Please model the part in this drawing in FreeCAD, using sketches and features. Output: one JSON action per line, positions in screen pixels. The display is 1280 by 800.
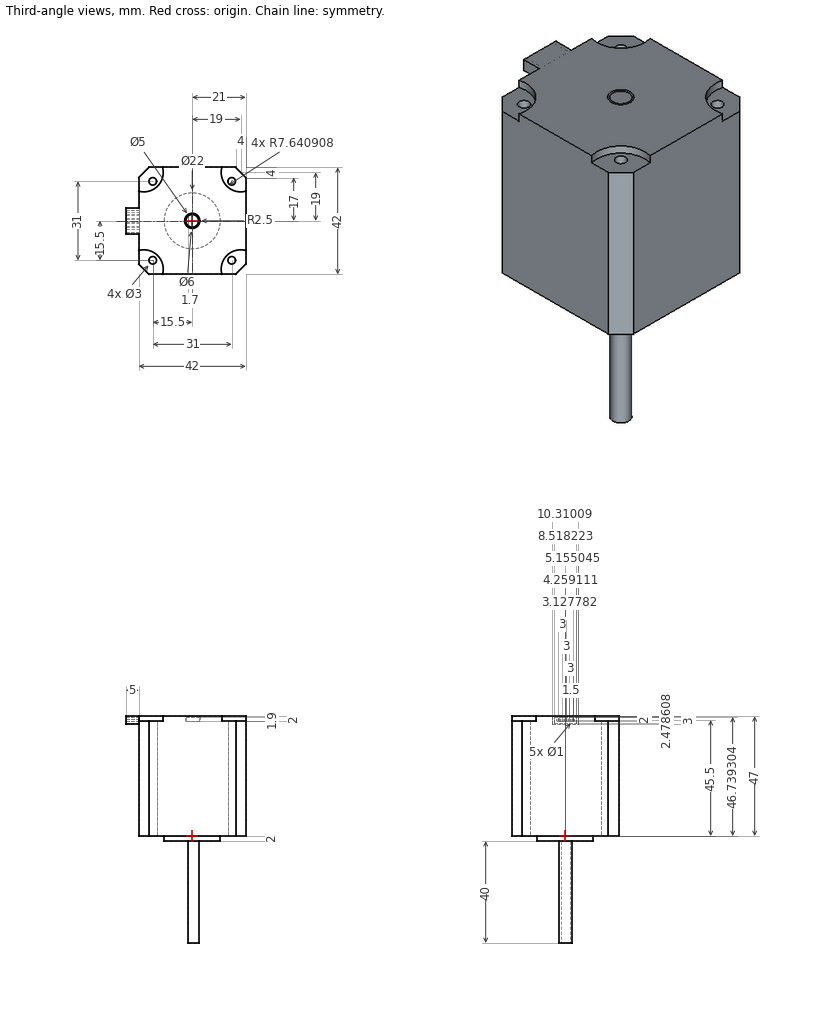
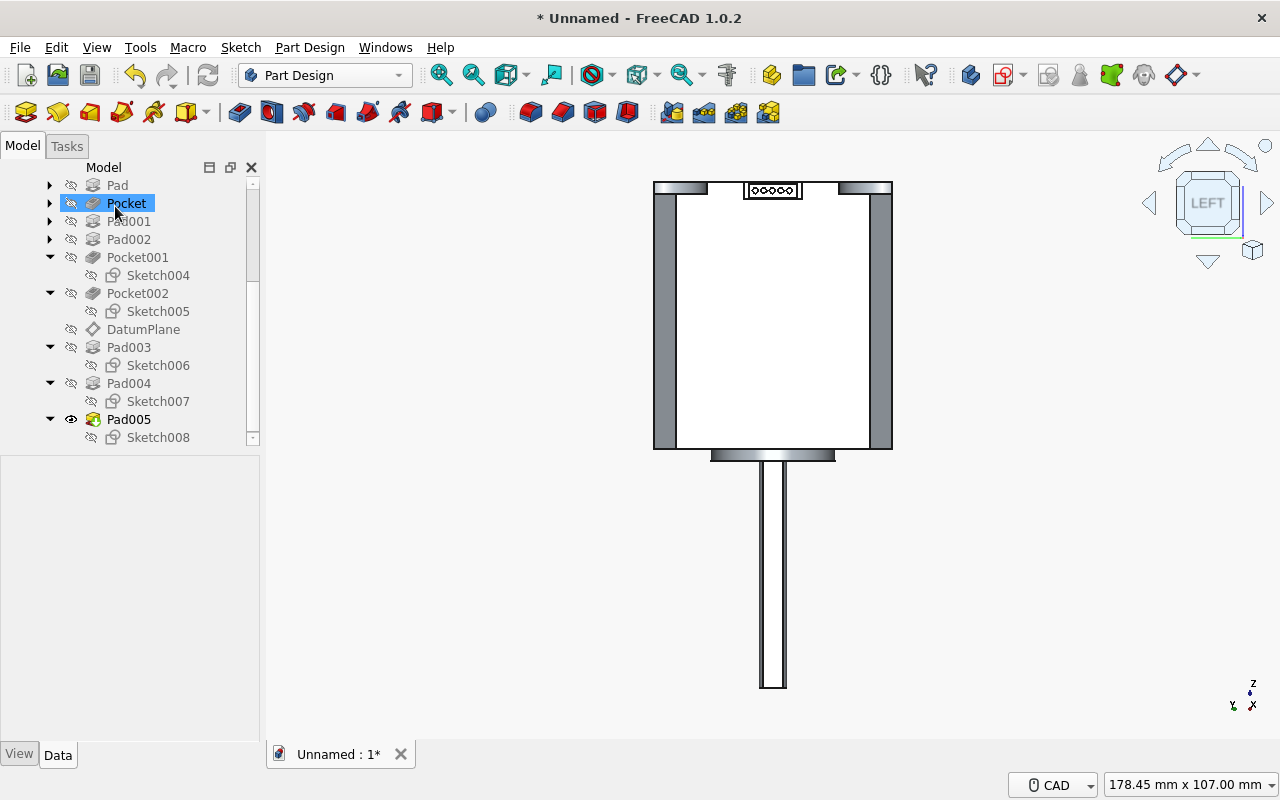
{"action": "key", "text": "0"}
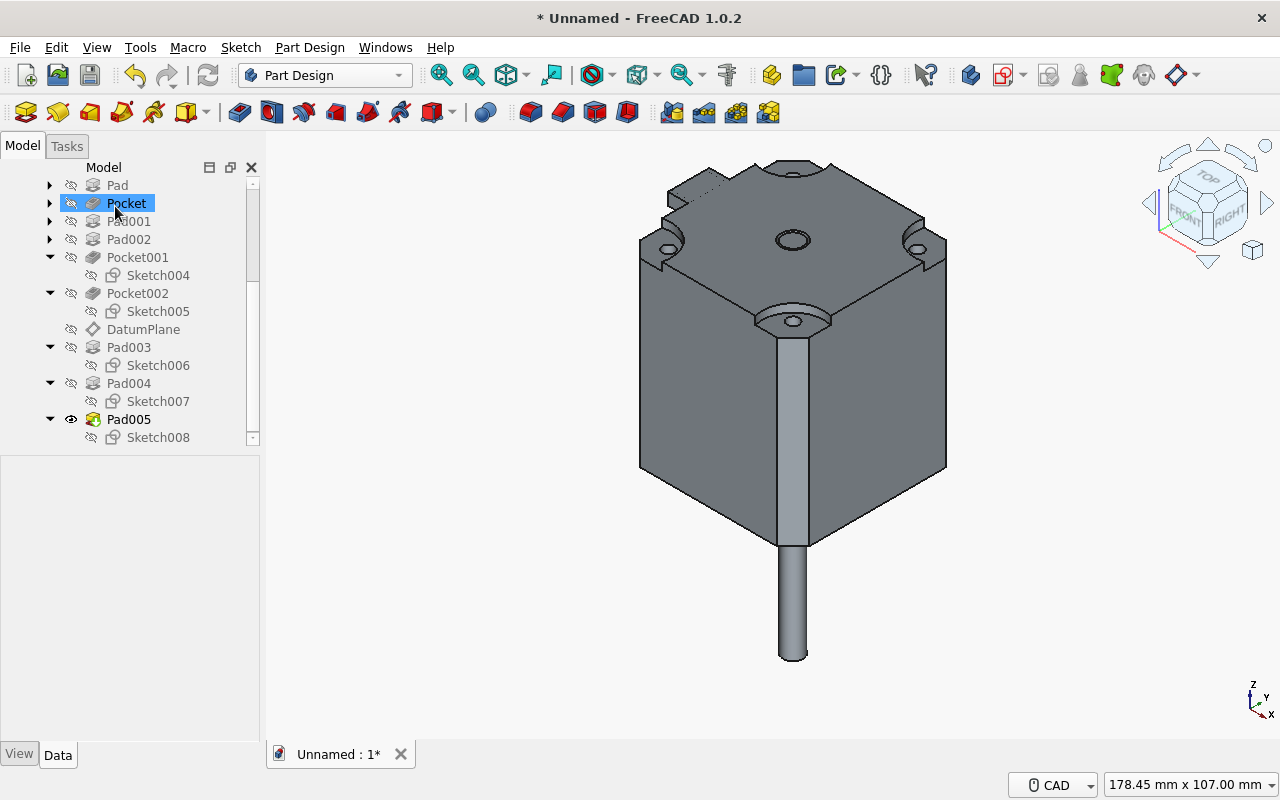
{"action": "left_click", "coordinate": [442, 76]}